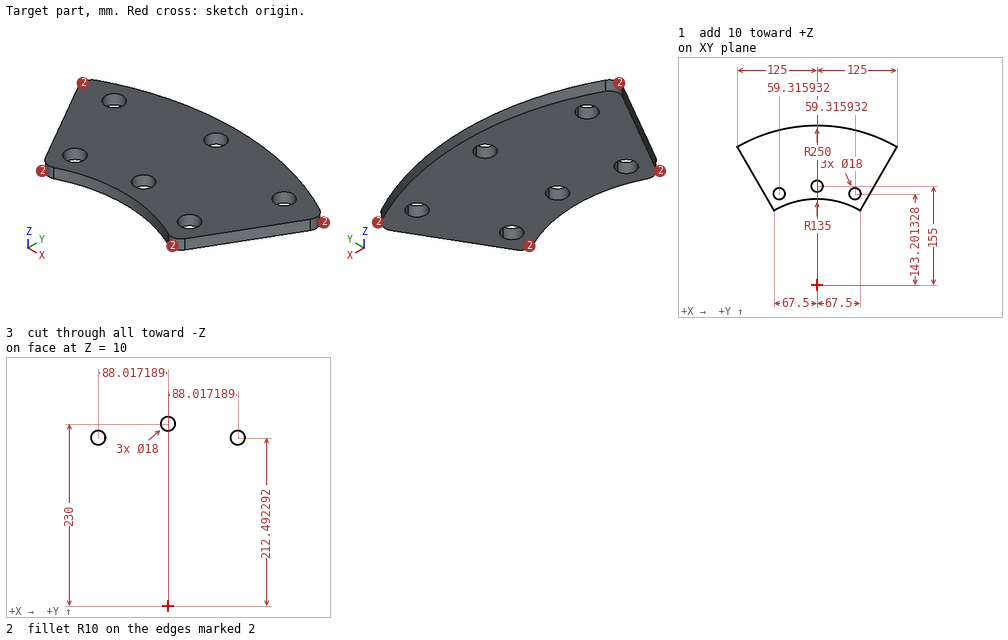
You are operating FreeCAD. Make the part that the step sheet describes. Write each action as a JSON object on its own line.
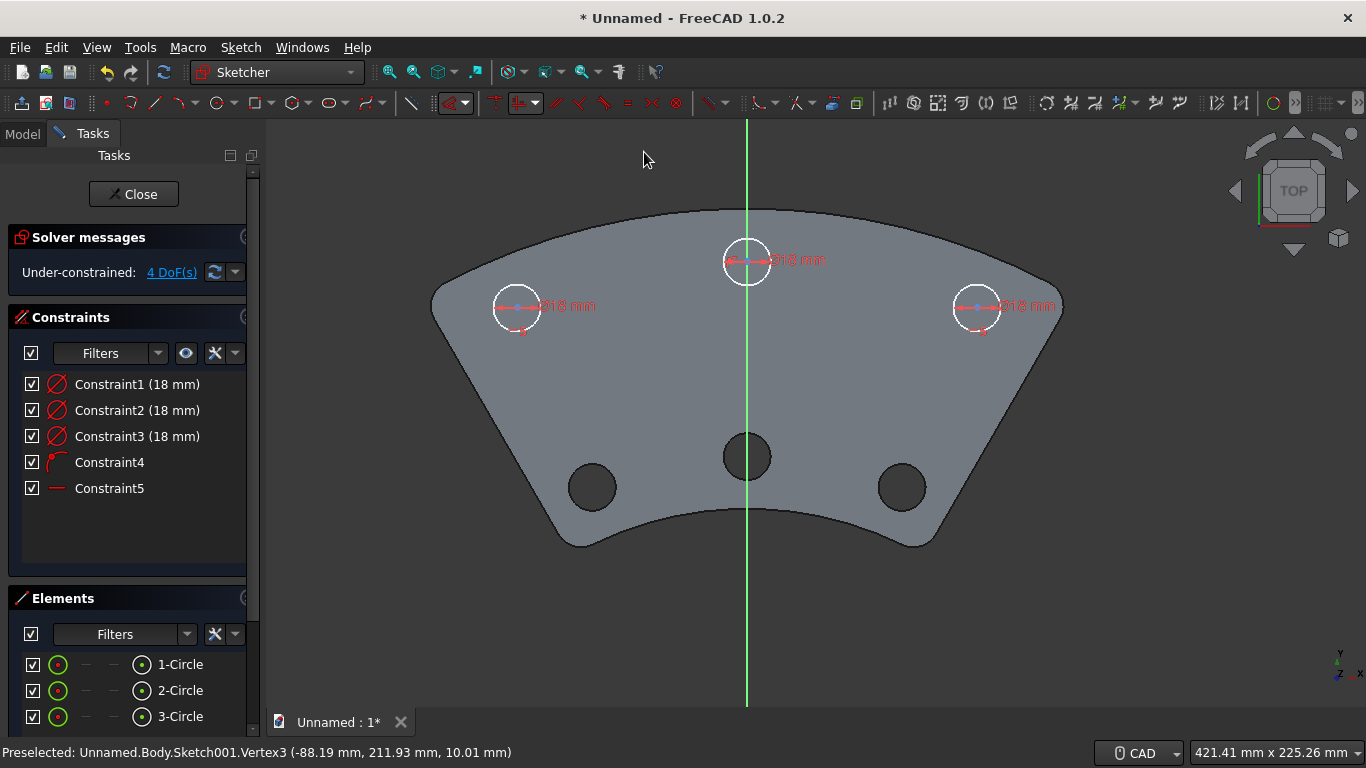
{"action": "left_click", "coordinate": [747, 262]}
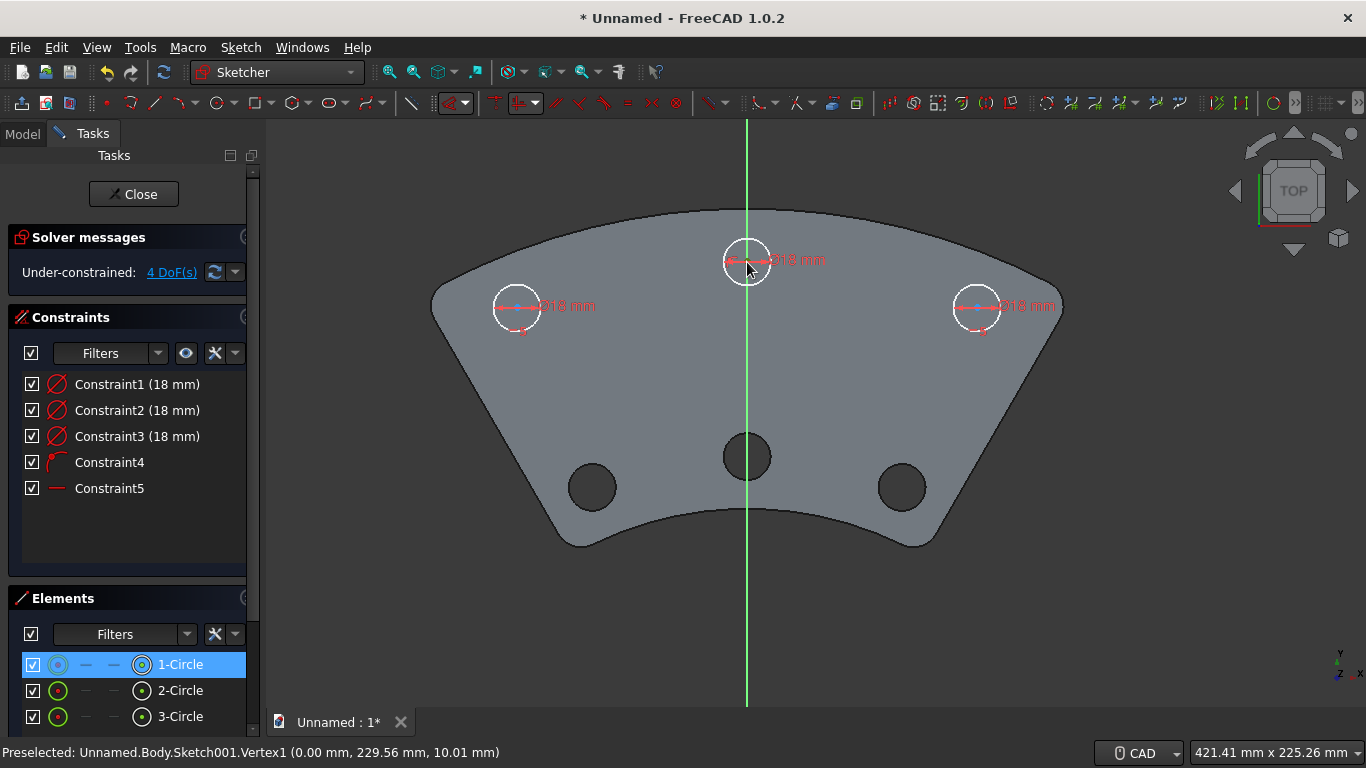
{"action": "key", "text": "i"}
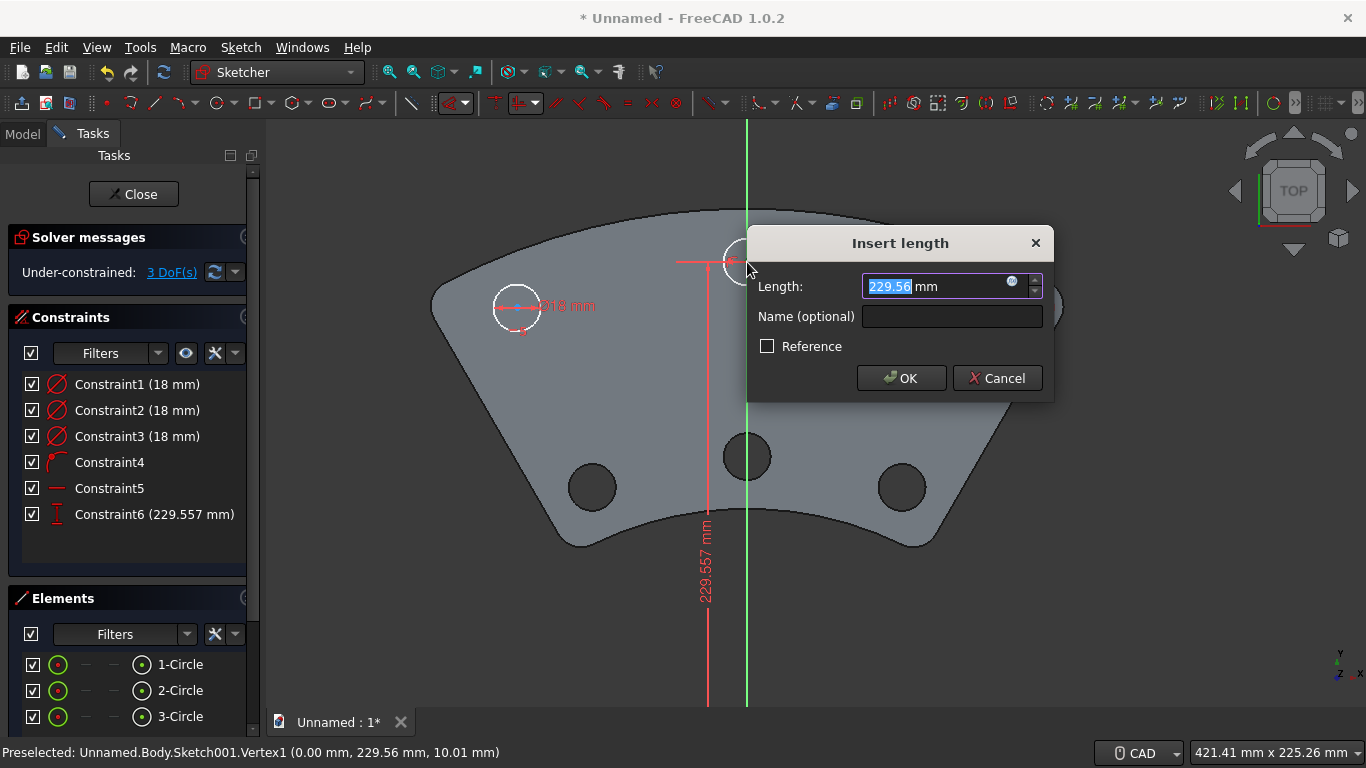
{"action": "type", "text": "230"}
{"action": "key", "text": "Return"}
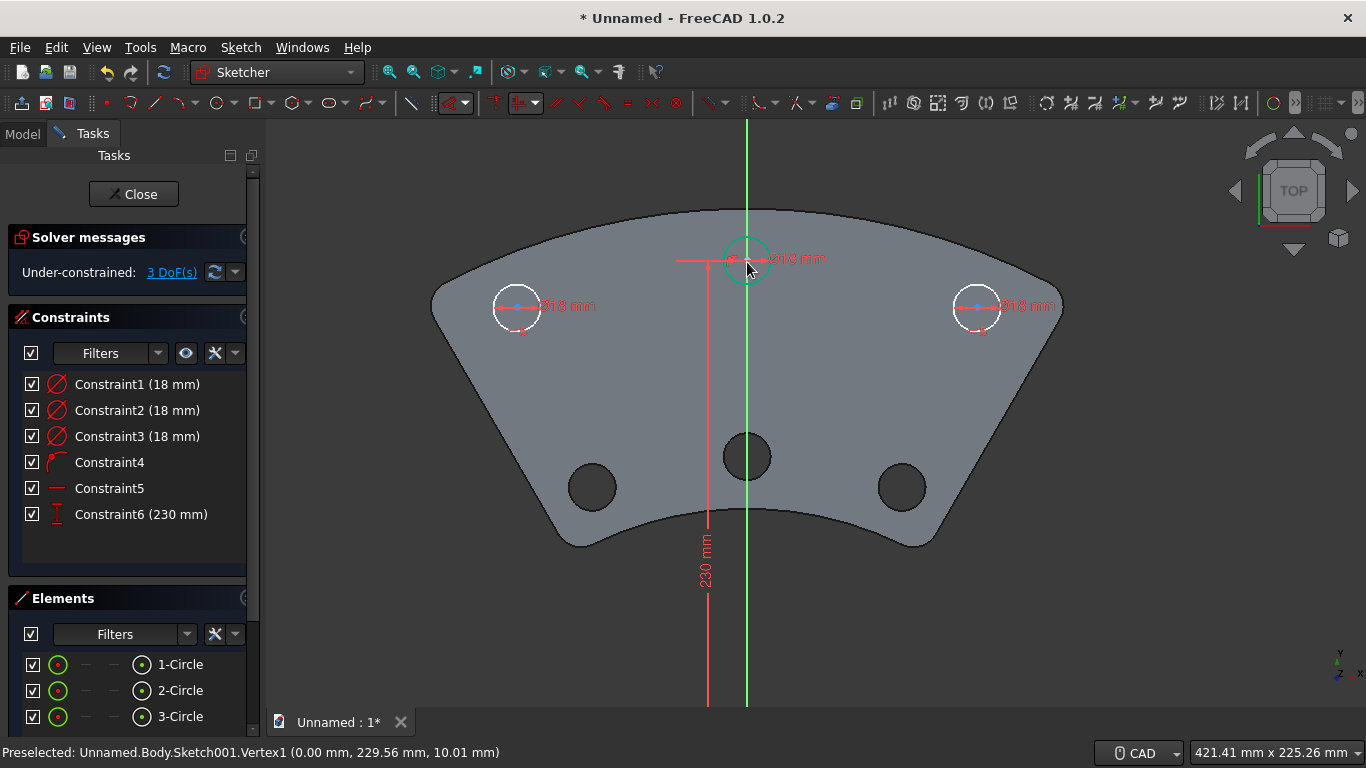
{"action": "left_click", "coordinate": [977, 308]}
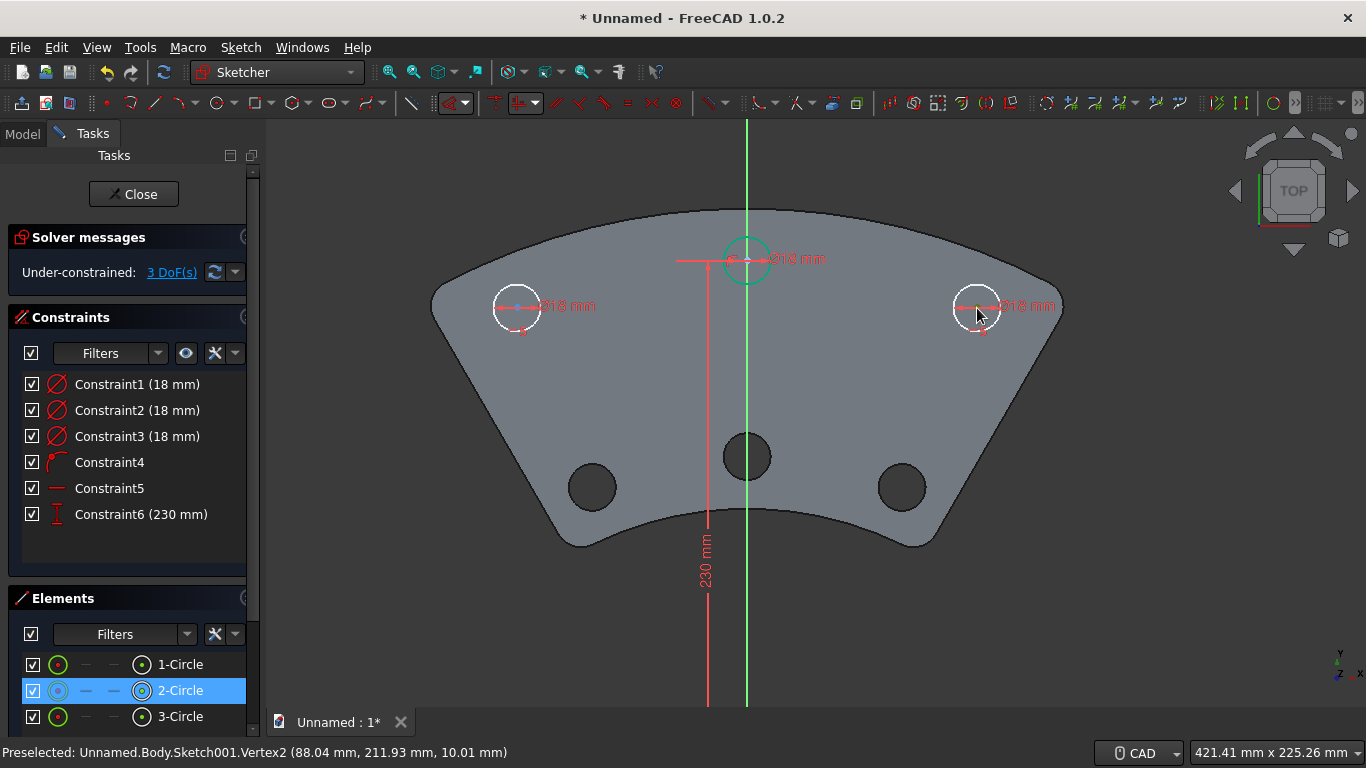
{"action": "key", "text": "l"}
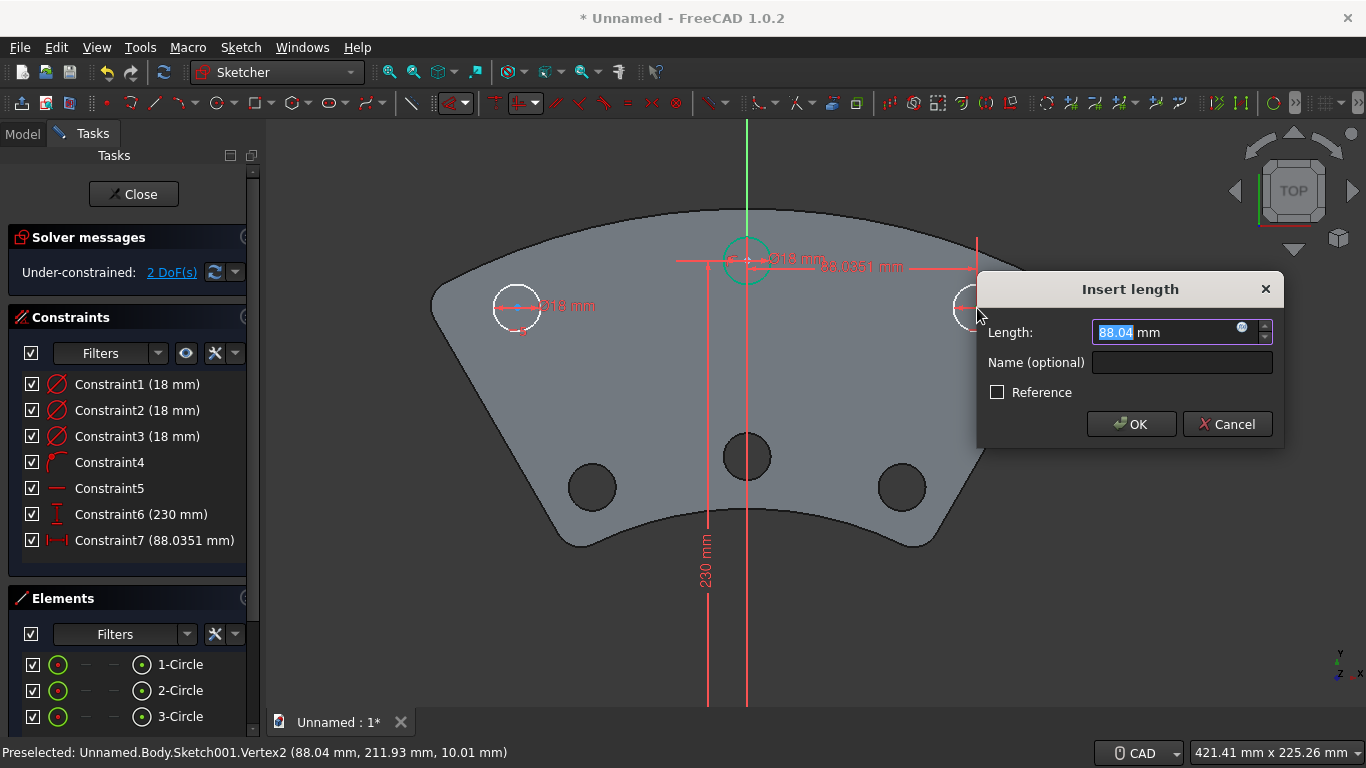
{"action": "type", "text": "88.017189"}
{"action": "key", "text": "Return"}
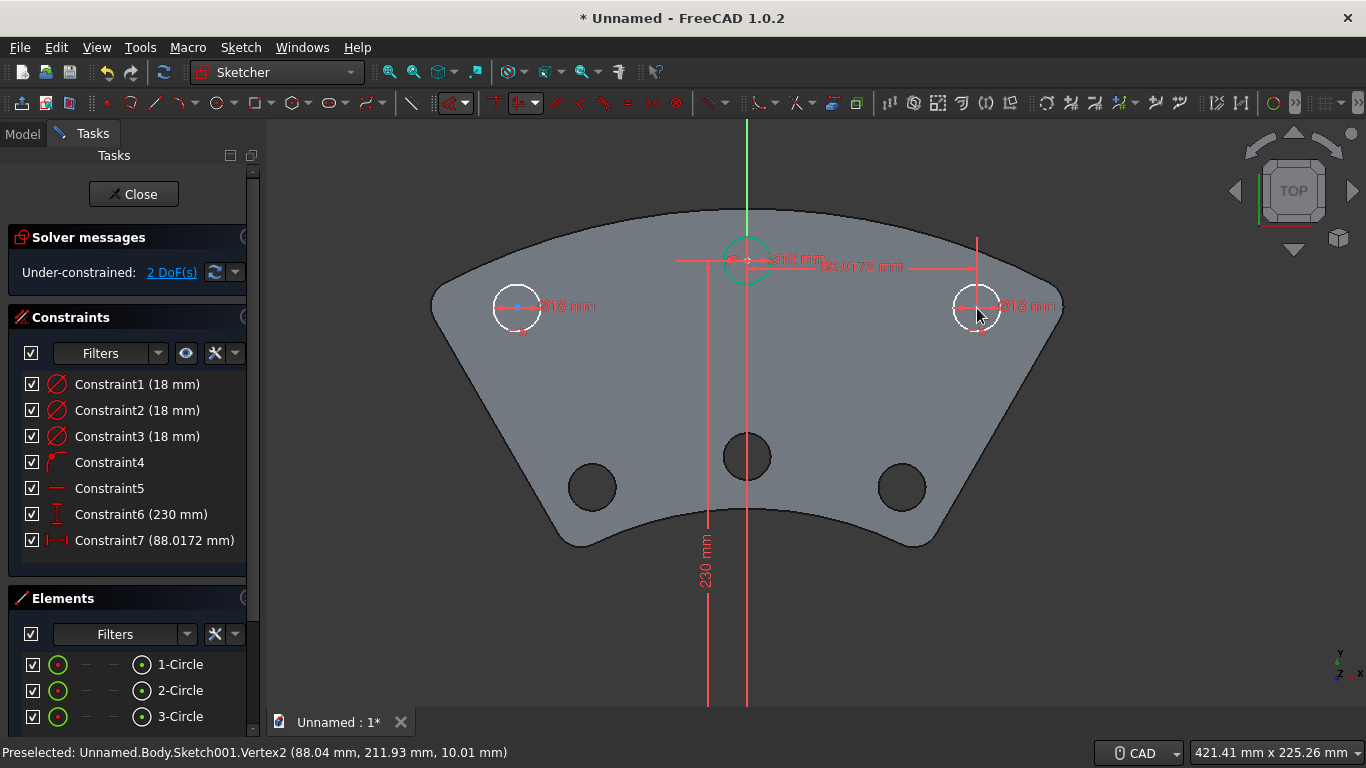
{"action": "left_click", "coordinate": [517, 308]}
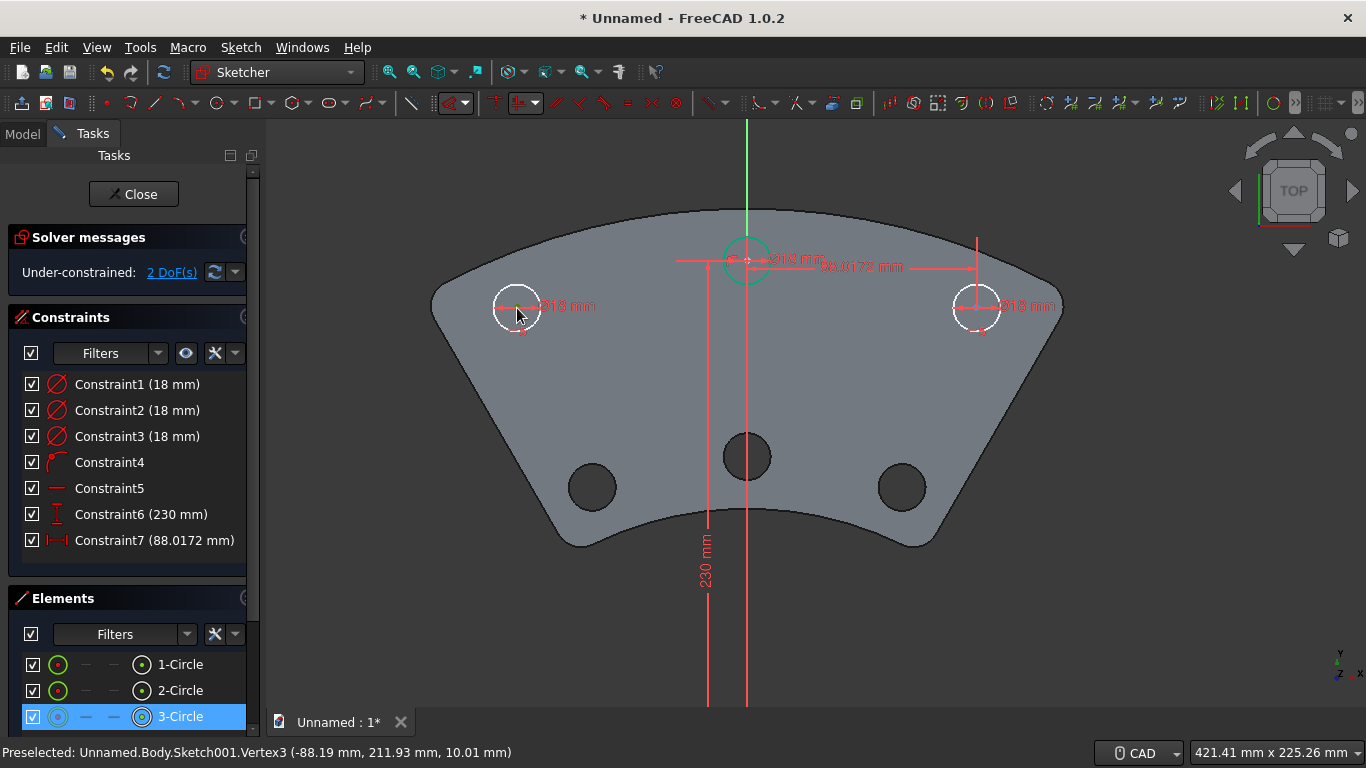
{"action": "left_click", "coordinate": [468, 104]}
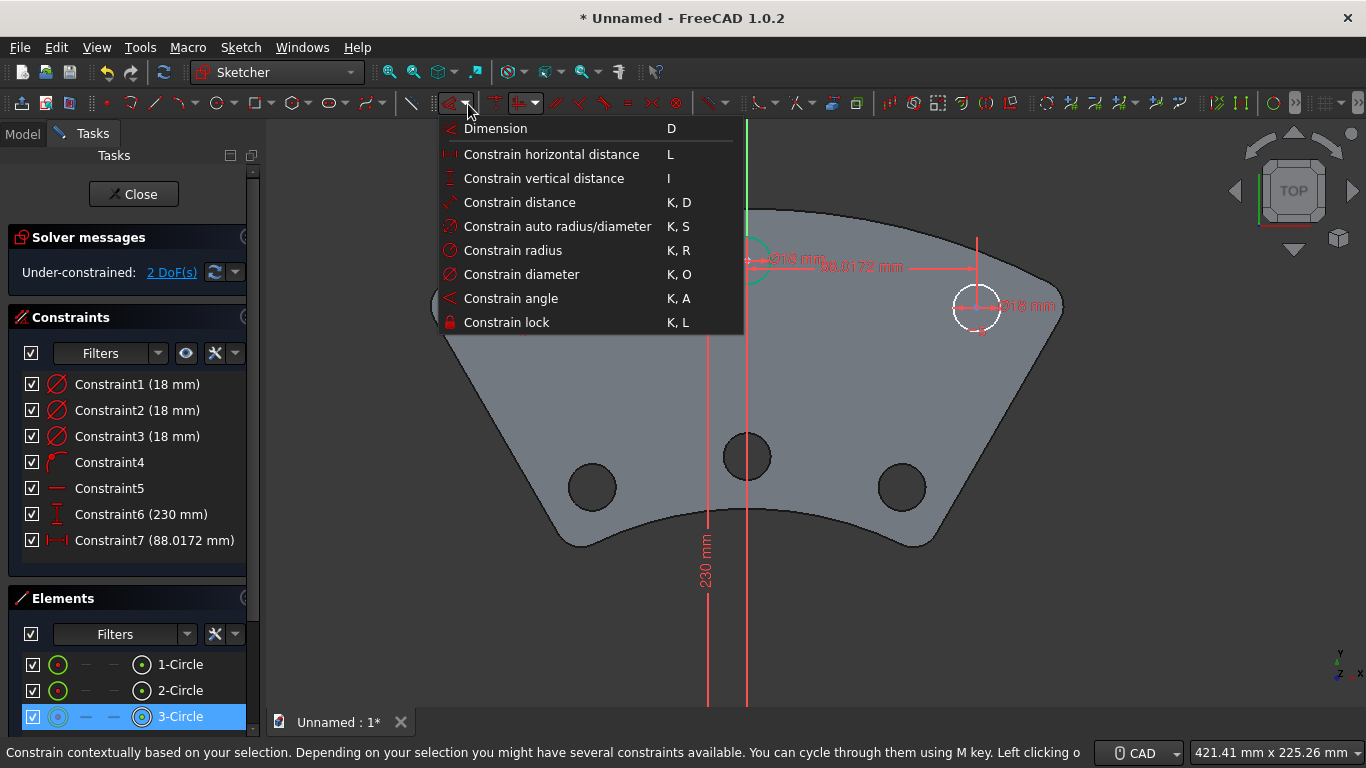
{"action": "left_click", "coordinate": [591, 154]}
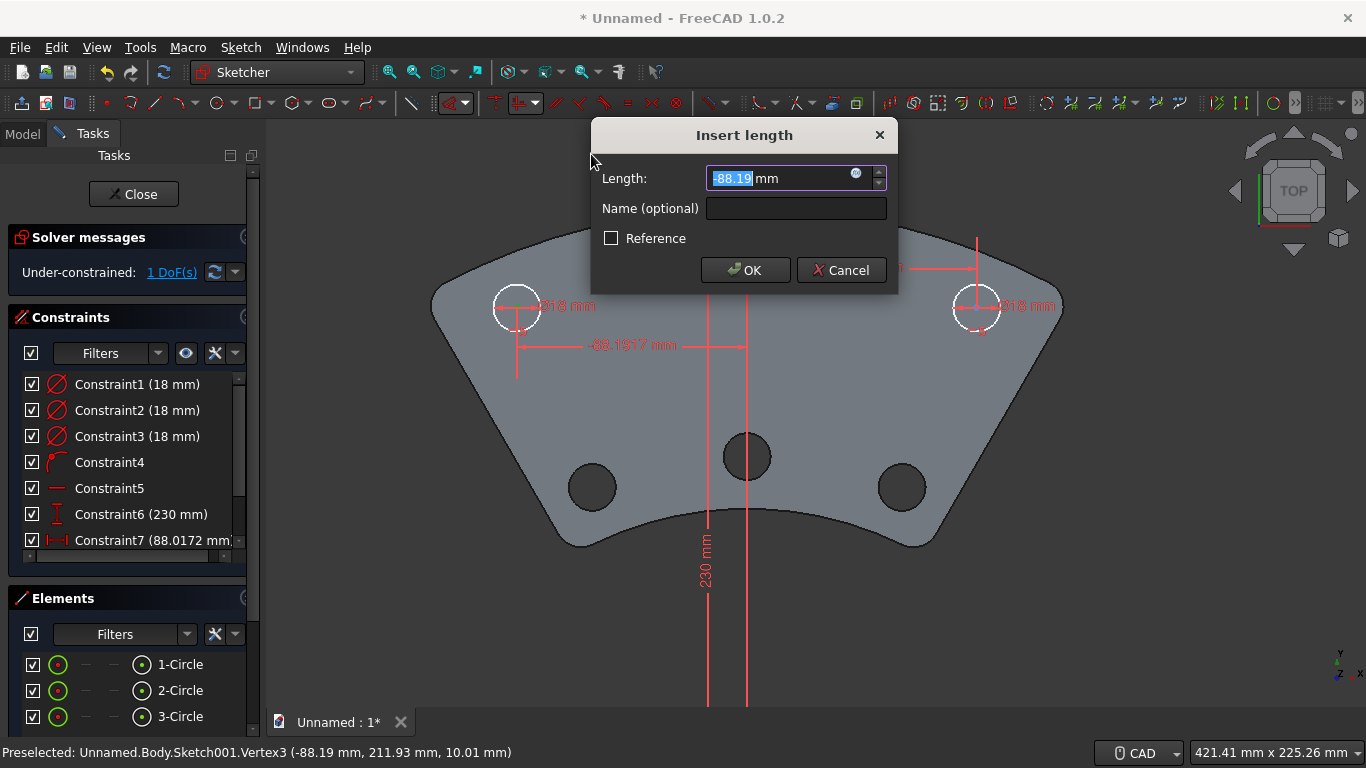
{"action": "type", "text": "-88.017189"}
{"action": "key", "text": "Return"}